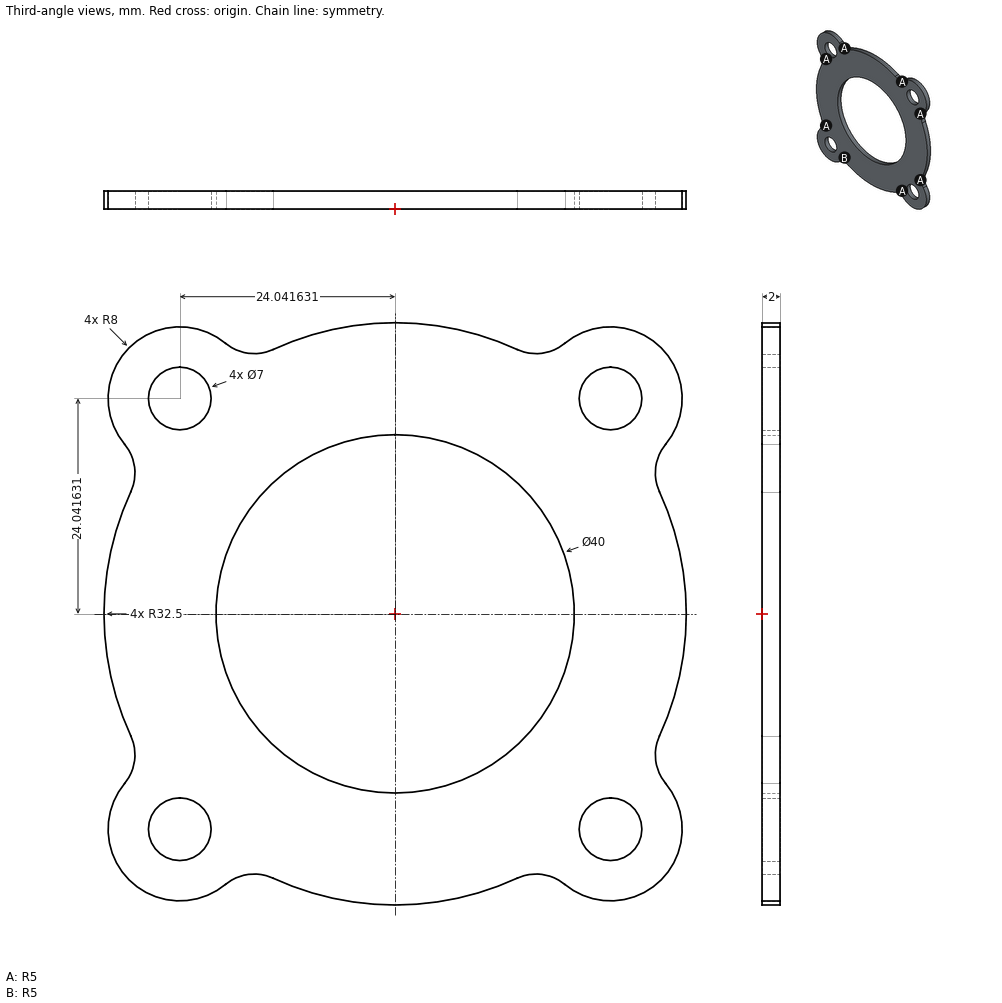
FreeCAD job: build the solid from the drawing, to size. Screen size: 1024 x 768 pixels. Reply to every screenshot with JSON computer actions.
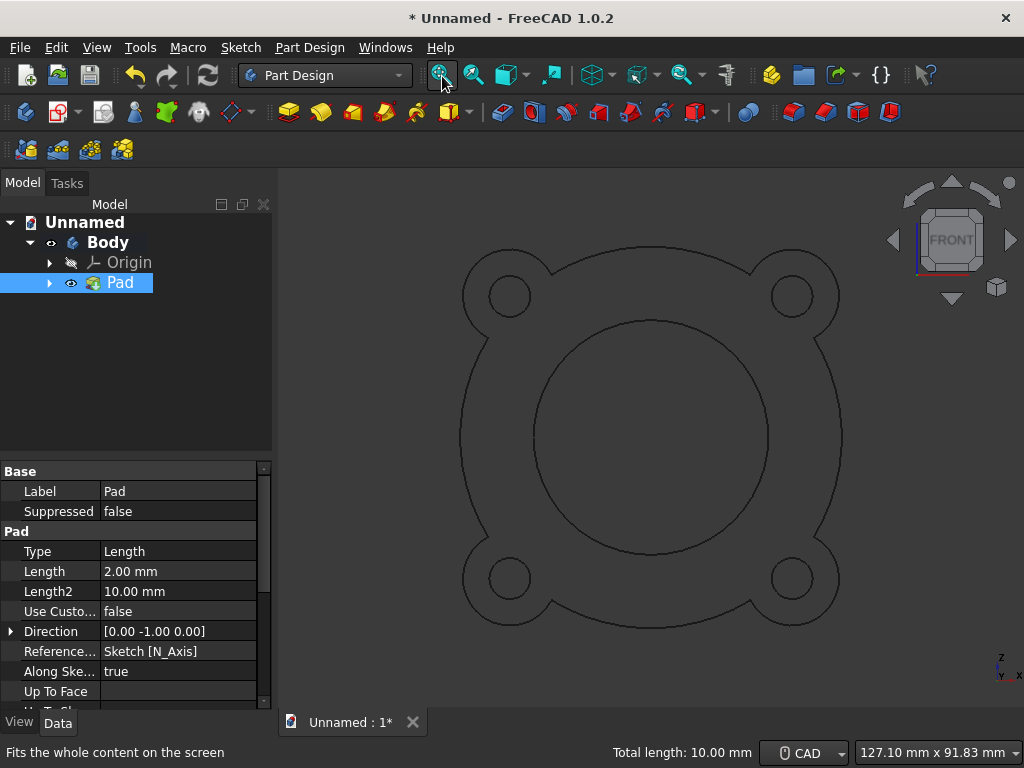
{"action": "scroll", "coordinate": [814, 337], "scroll_direction": "up", "scroll_amount": 7}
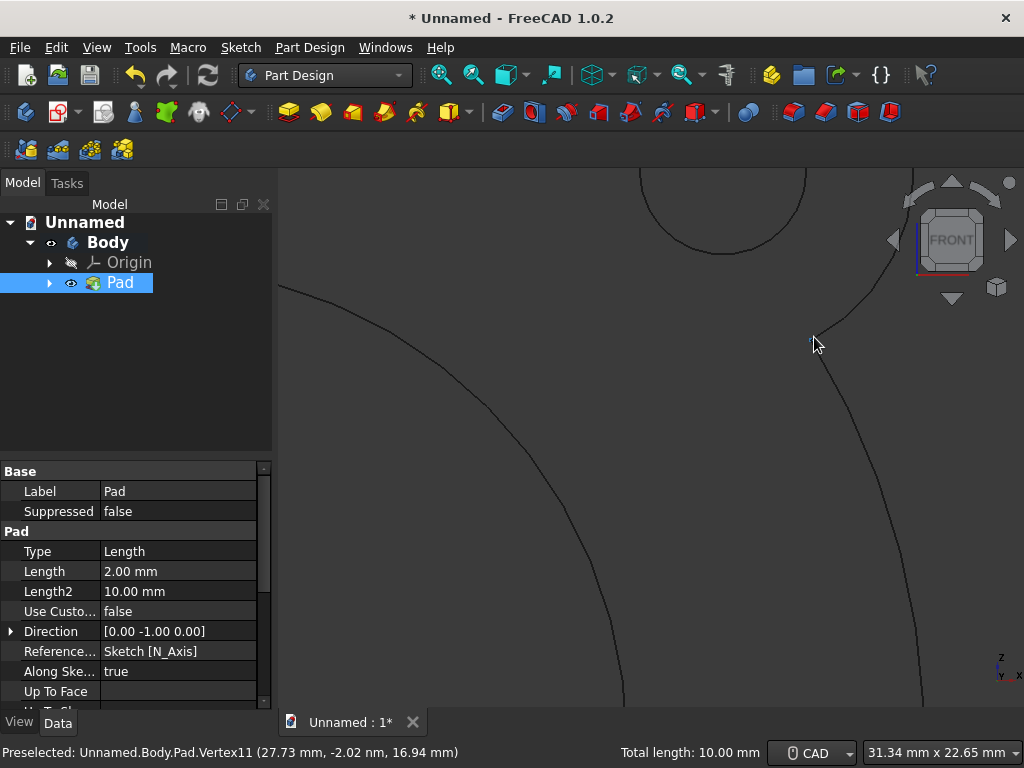
{"action": "left_click", "coordinate": [442, 76]}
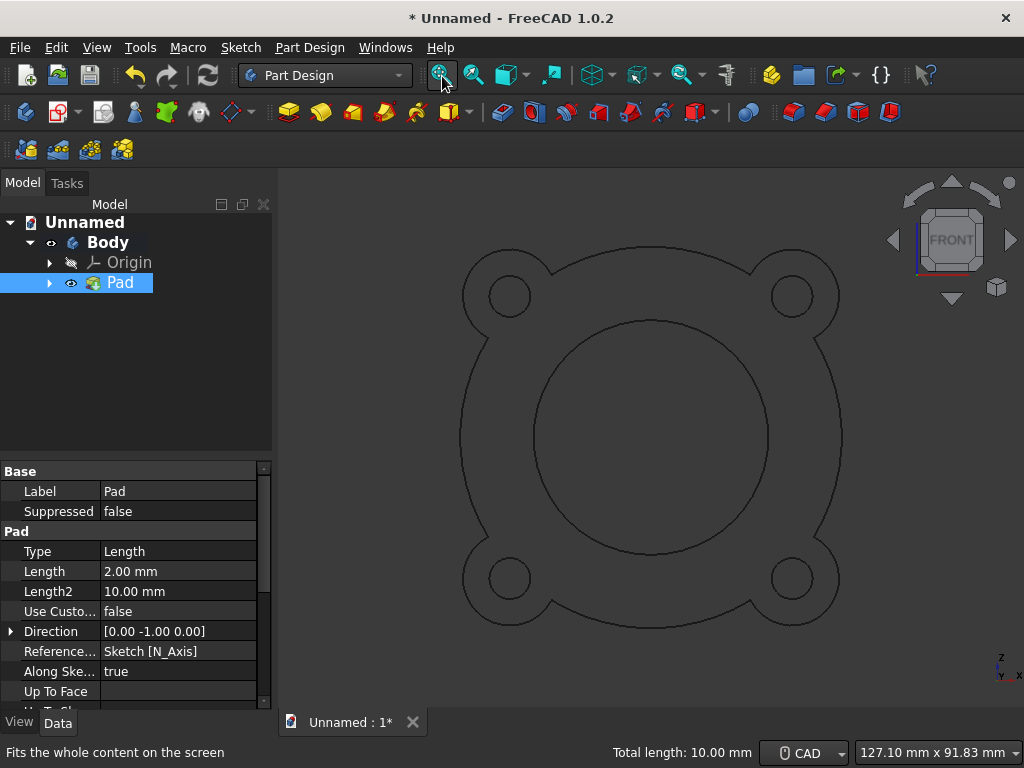
{"action": "key", "text": "3"}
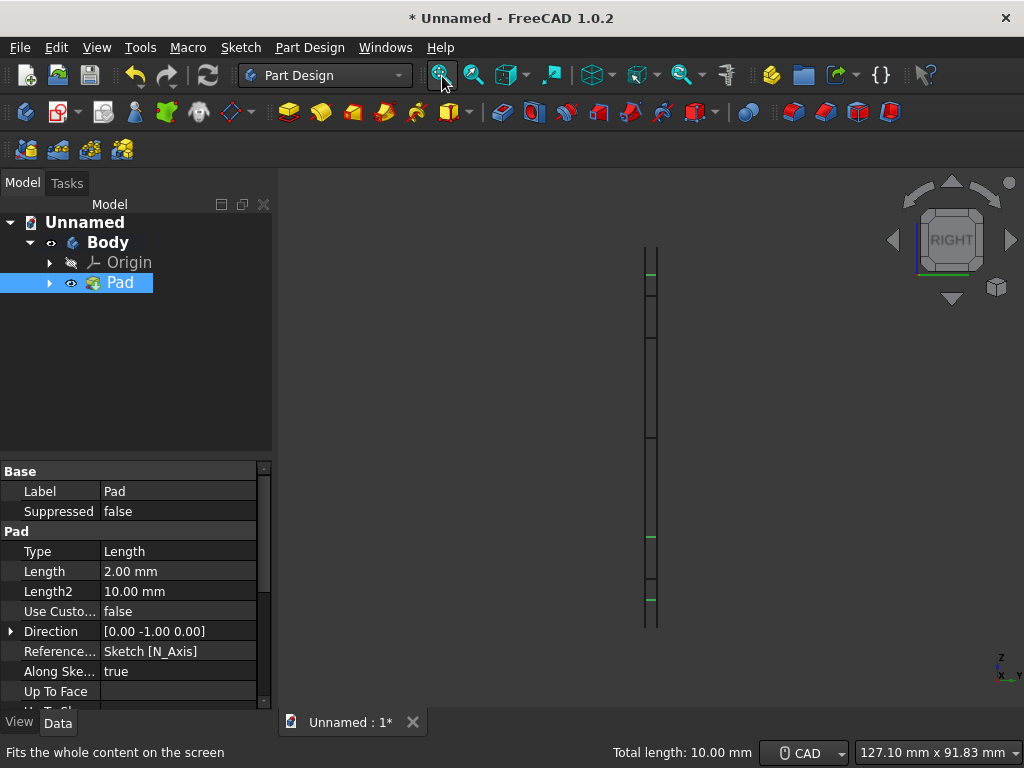
{"action": "scroll", "coordinate": [651, 337], "scroll_direction": "up", "scroll_amount": 7}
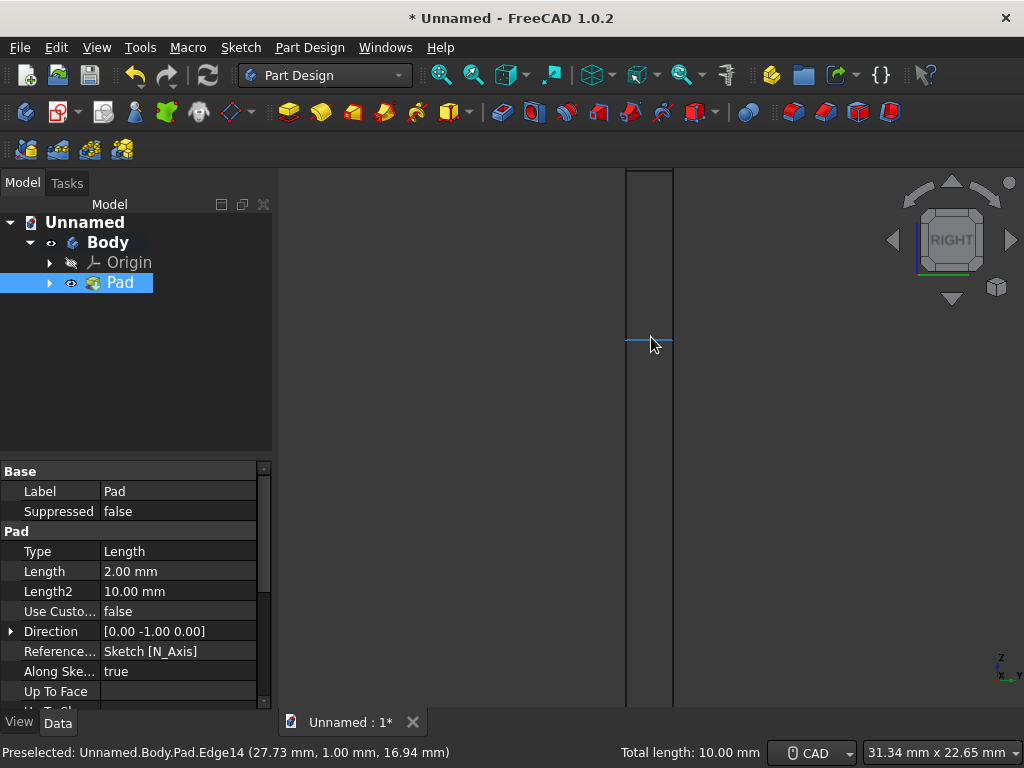
{"action": "left_click", "coordinate": [649, 339], "text": "ctrl"}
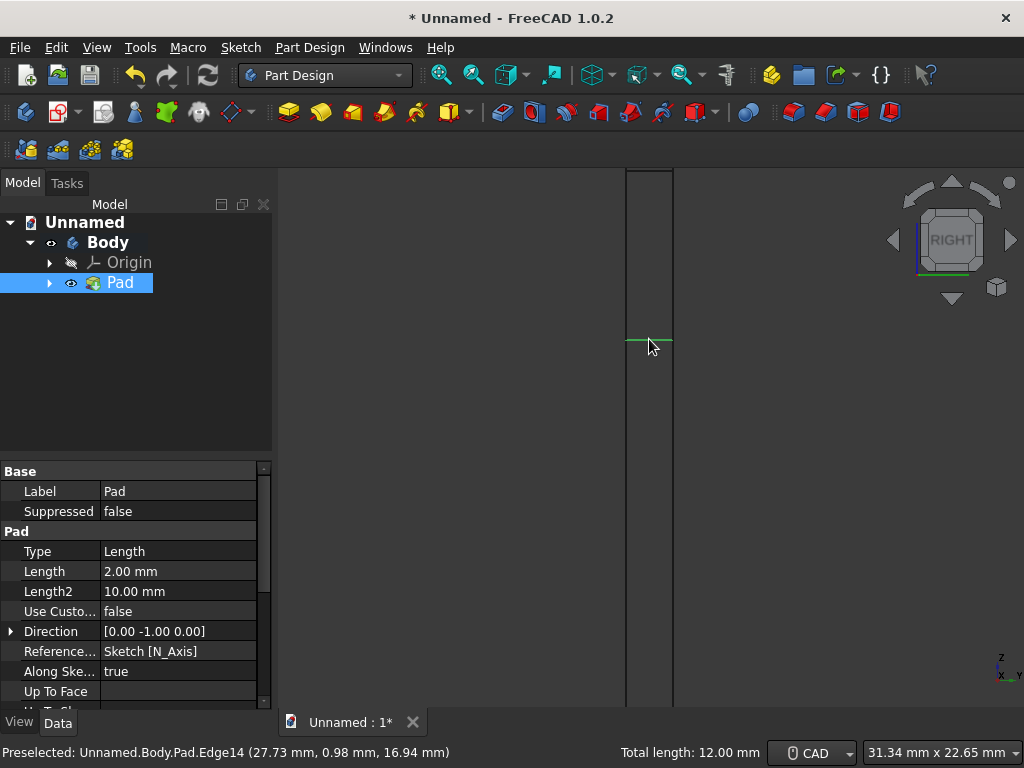
{"action": "left_click", "coordinate": [442, 76]}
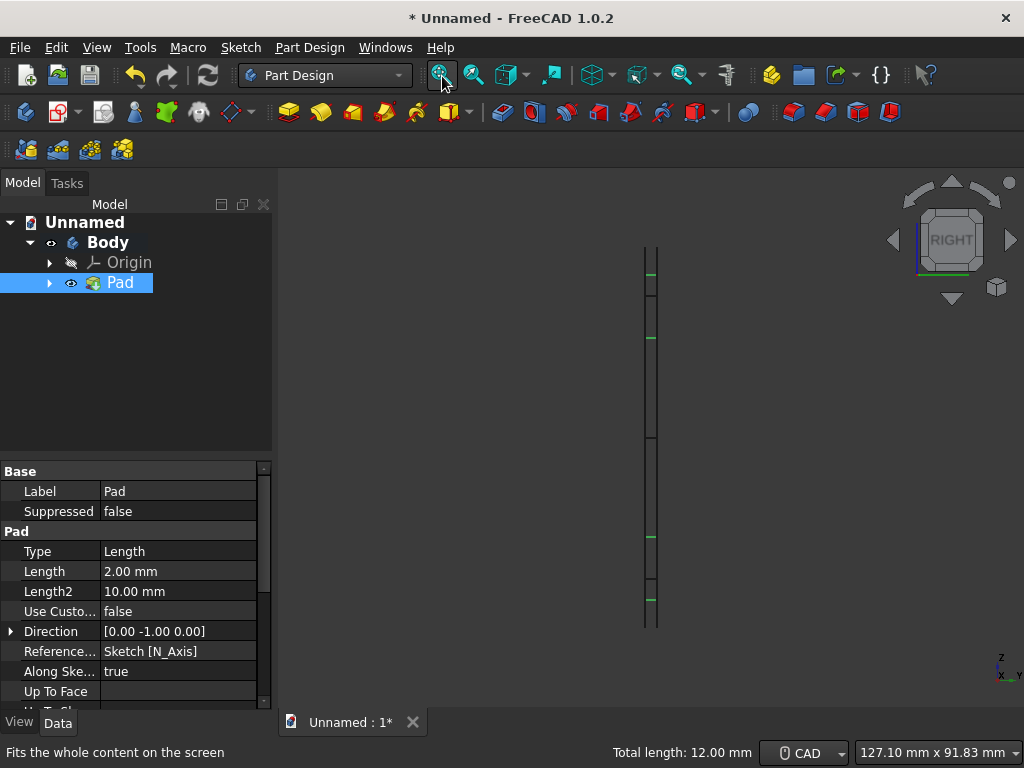
{"action": "key", "text": "5"}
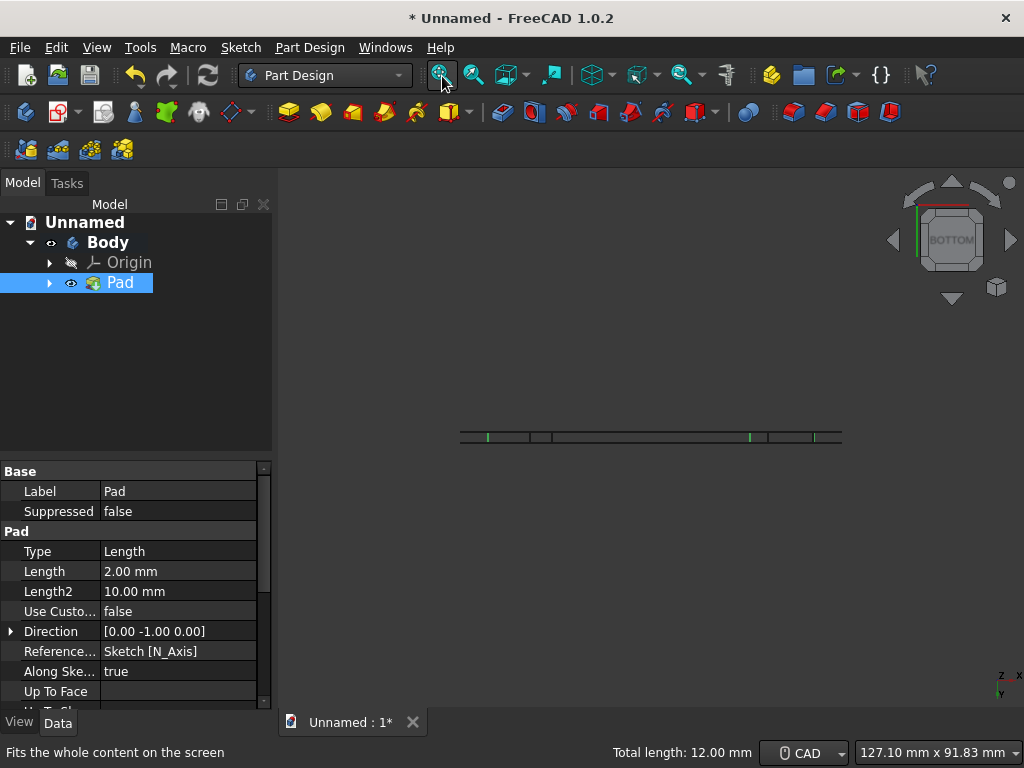
{"action": "scroll", "coordinate": [552, 436], "scroll_direction": "up", "scroll_amount": 7}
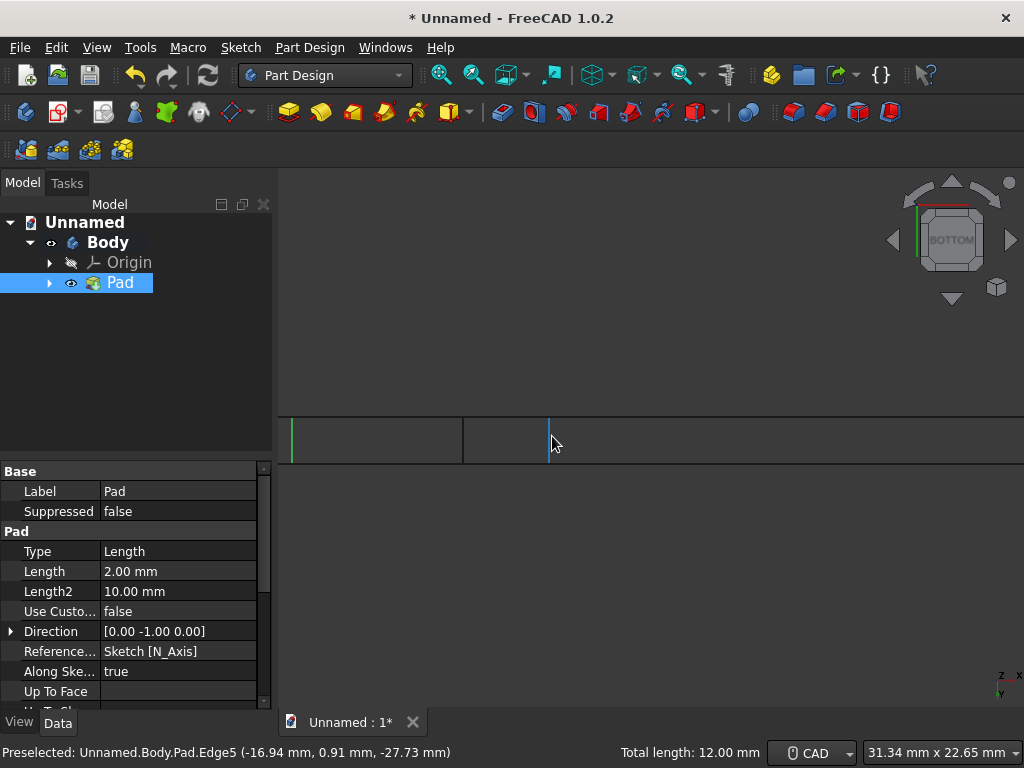
{"action": "left_click", "coordinate": [442, 76]}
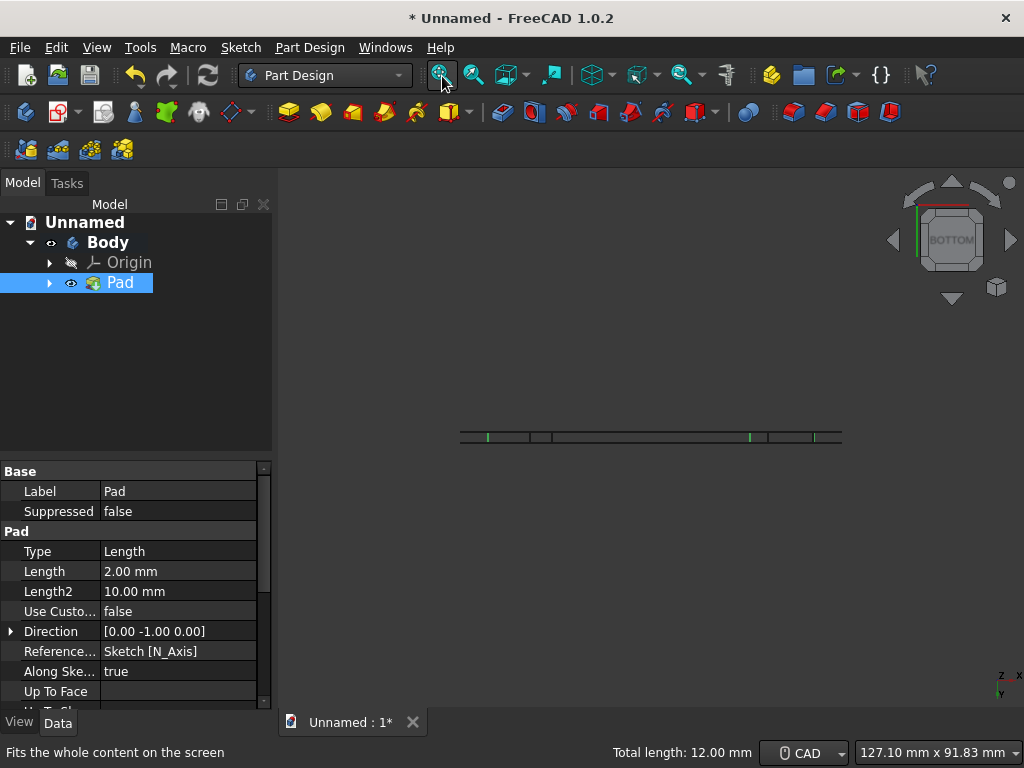
{"action": "key", "text": "4"}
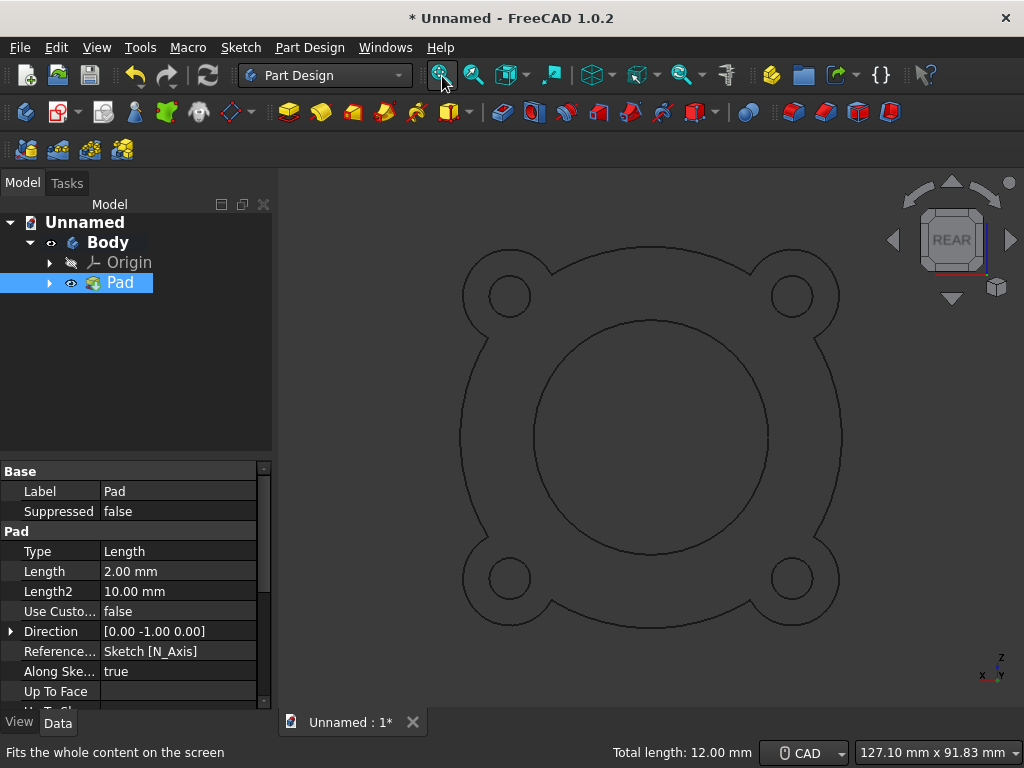
{"action": "scroll", "coordinate": [750, 274], "scroll_direction": "up", "scroll_amount": 7}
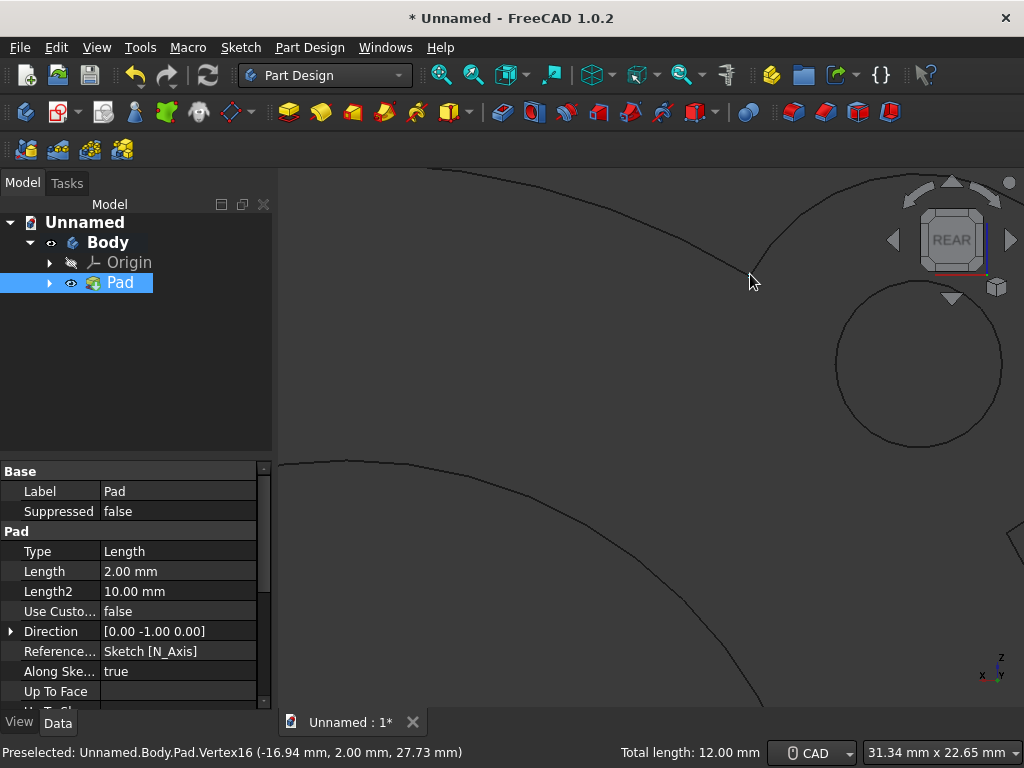
{"action": "left_click", "coordinate": [442, 76]}